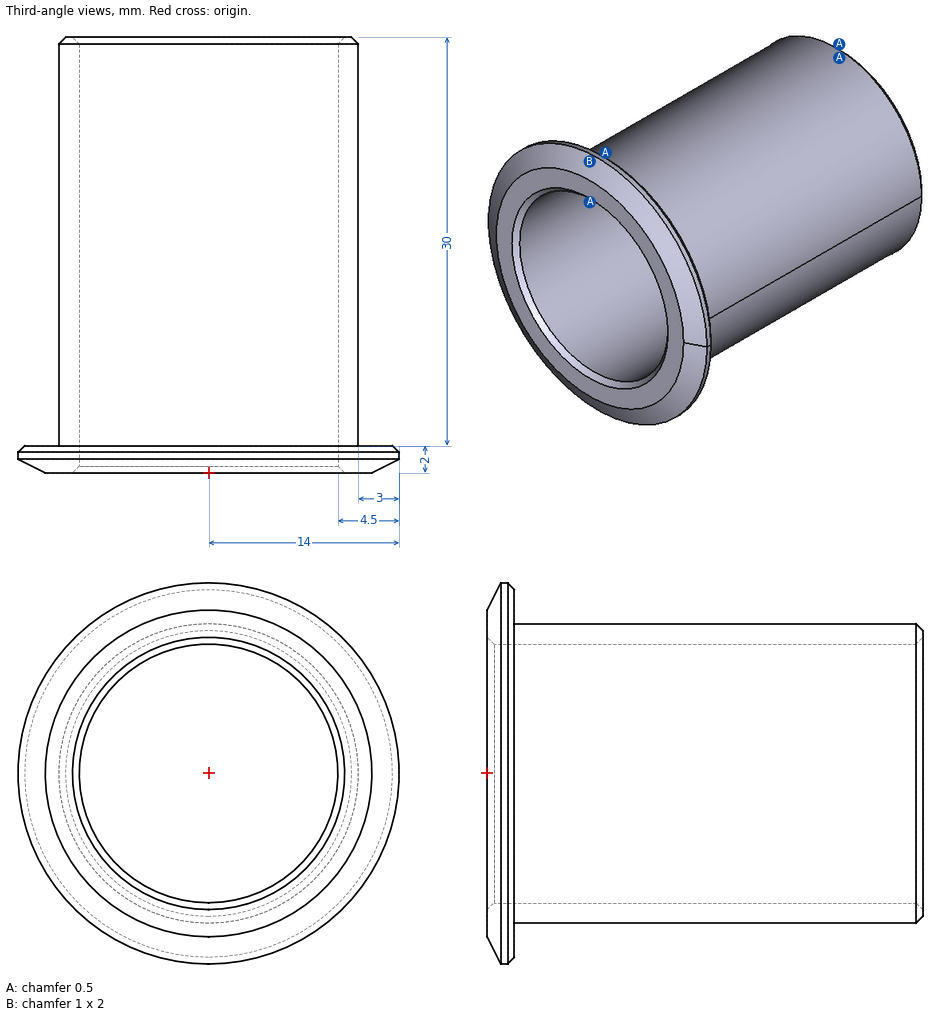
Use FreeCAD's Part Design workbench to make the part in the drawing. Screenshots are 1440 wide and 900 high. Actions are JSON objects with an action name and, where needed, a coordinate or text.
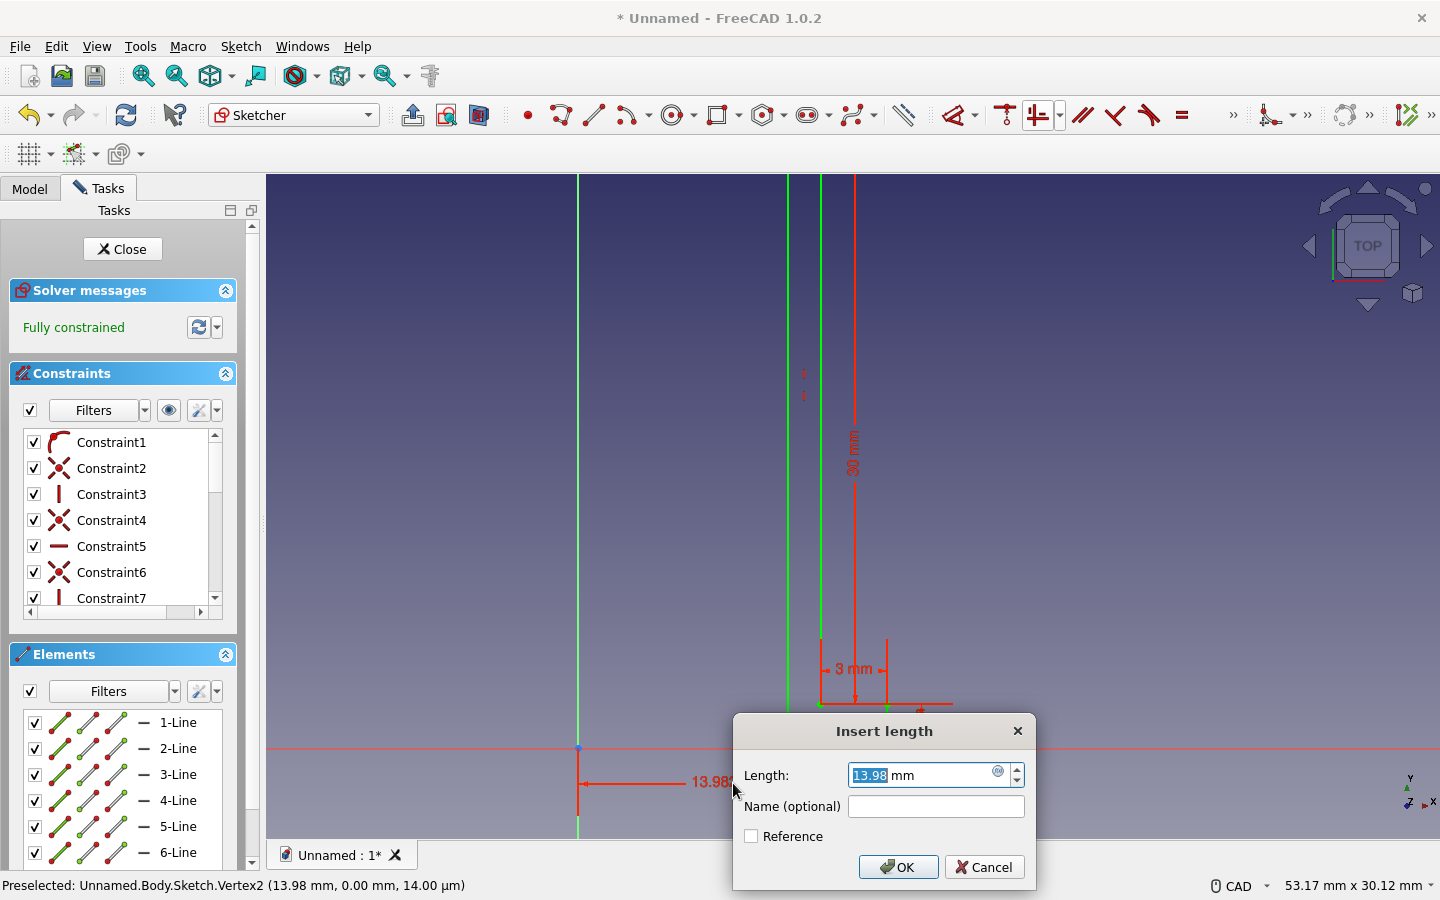
{"action": "type", "text": "14"}
{"action": "key", "text": "Return"}
{"action": "key", "text": "Escape"}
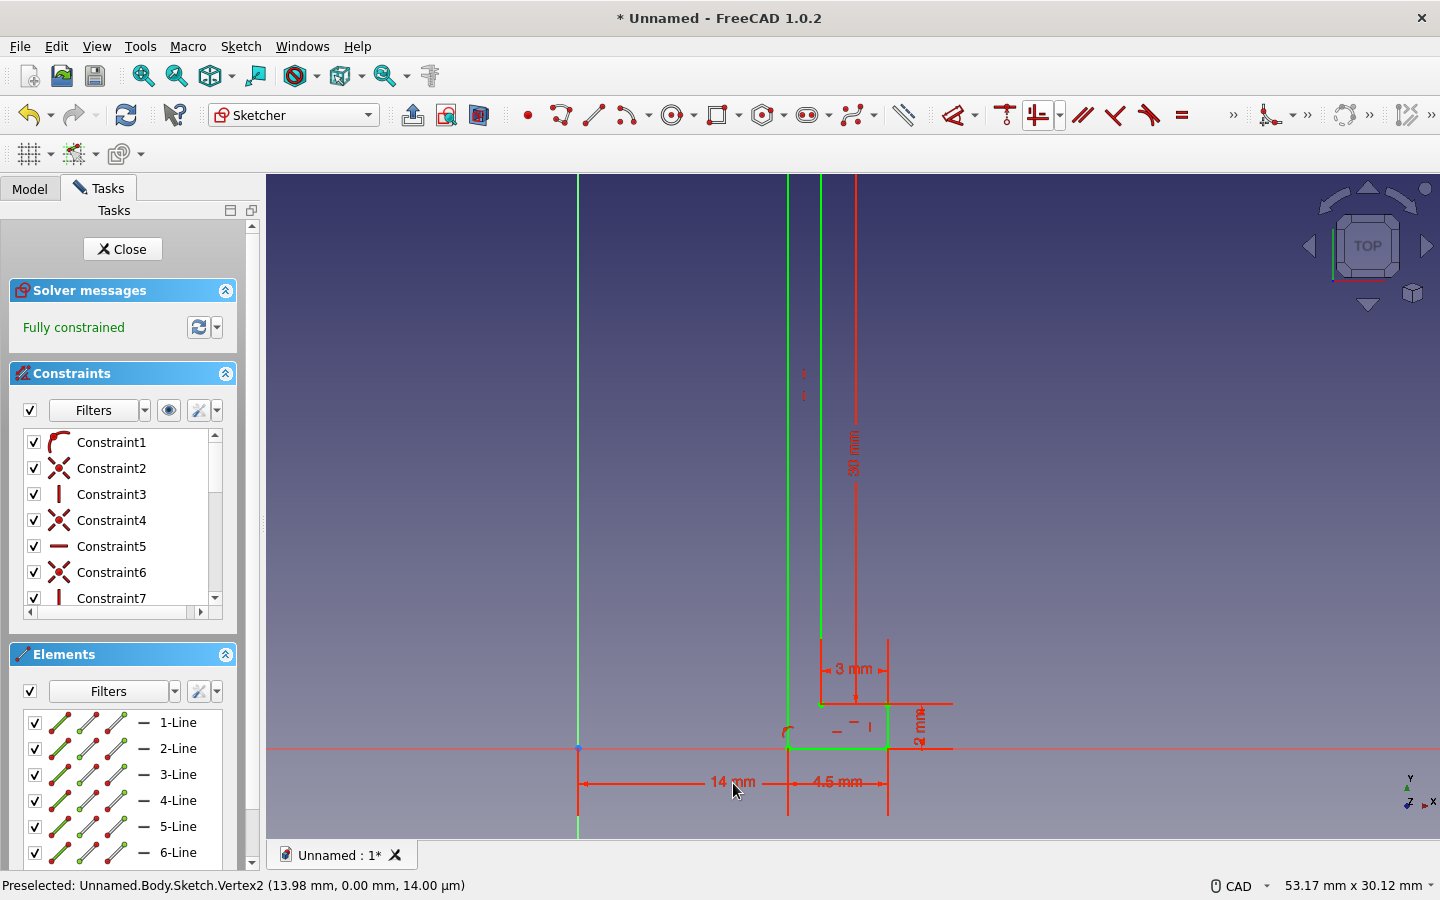
{"action": "left_click", "coordinate": [123, 249]}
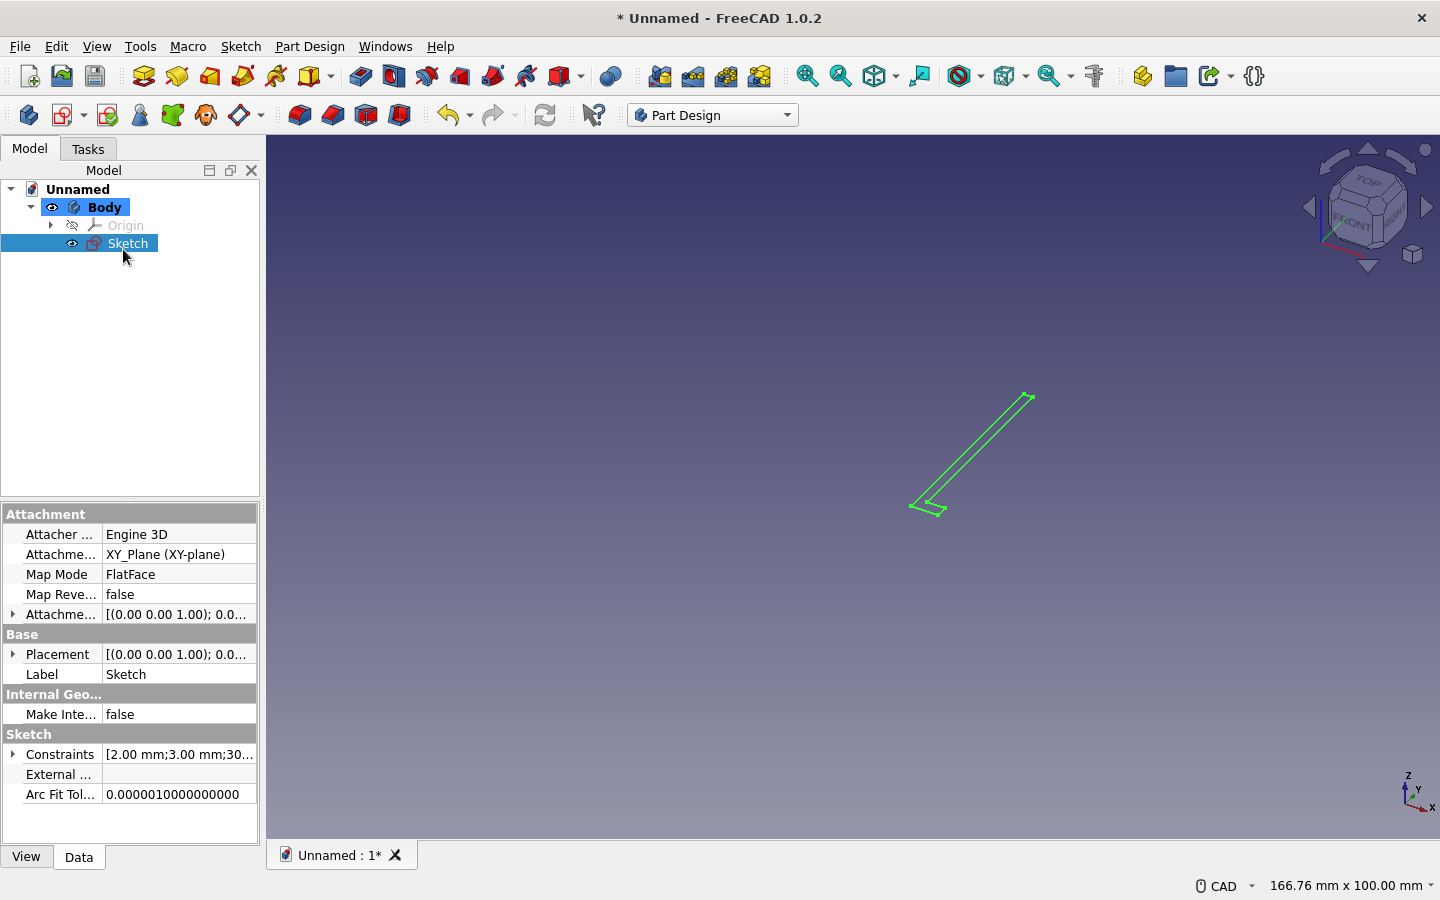
{"action": "left_click", "coordinate": [177, 76]}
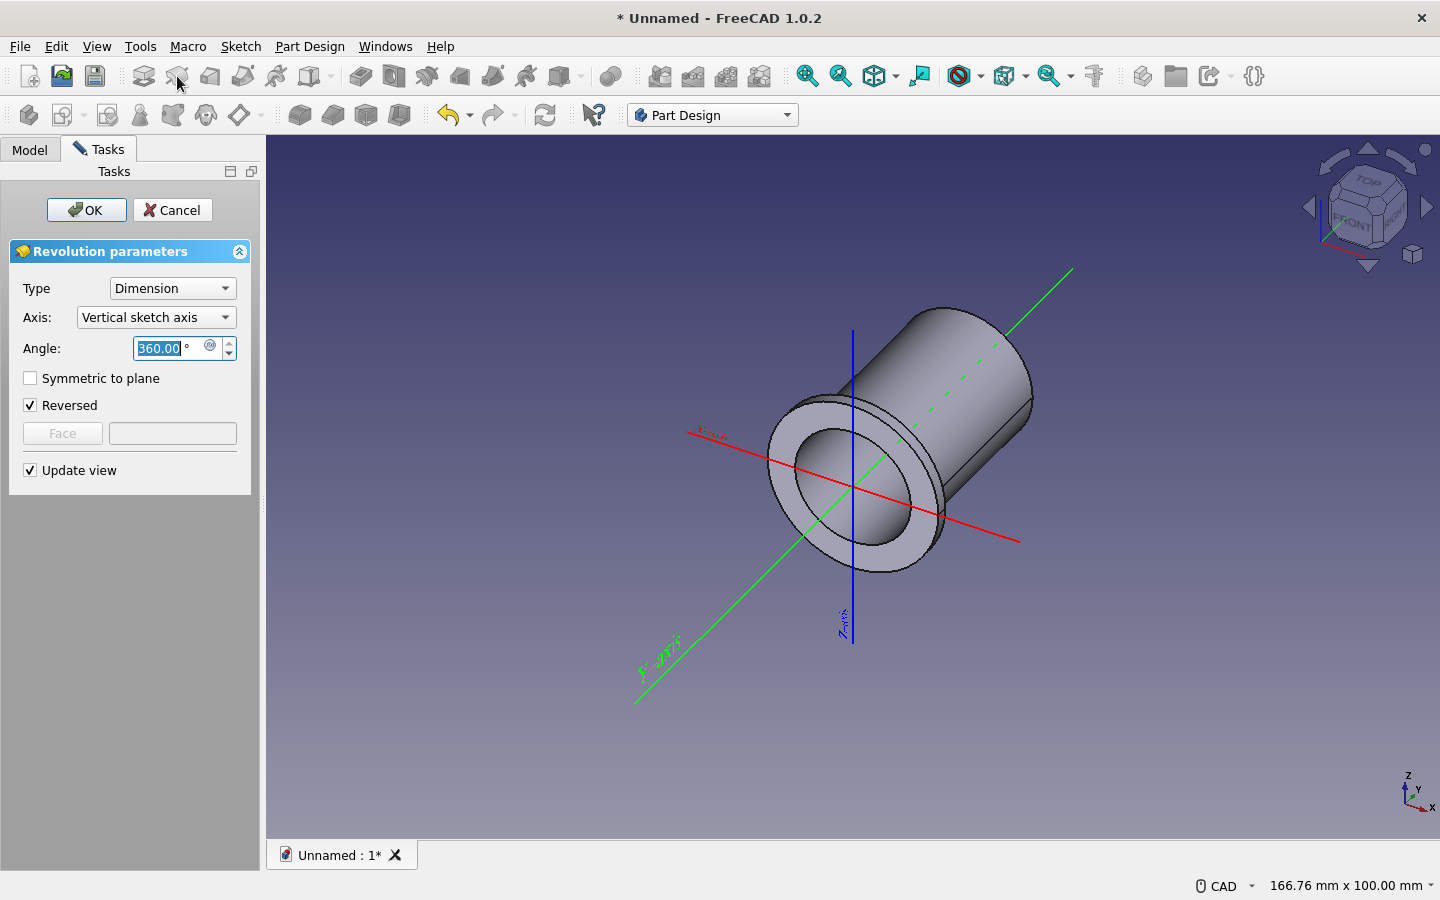
{"action": "left_click", "coordinate": [87, 210]}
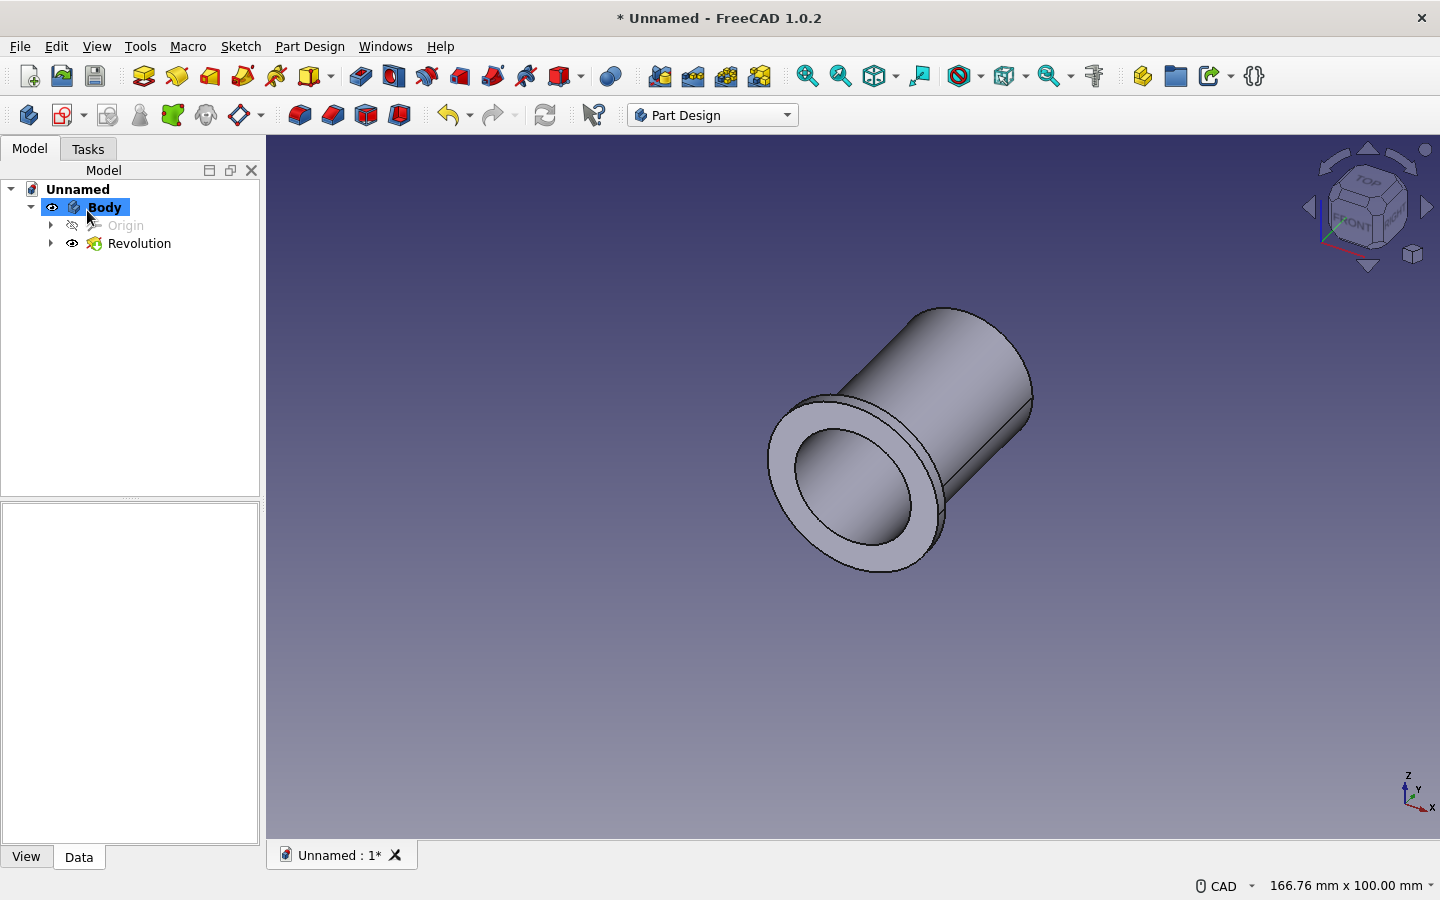
{"action": "left_click", "coordinate": [795, 467]}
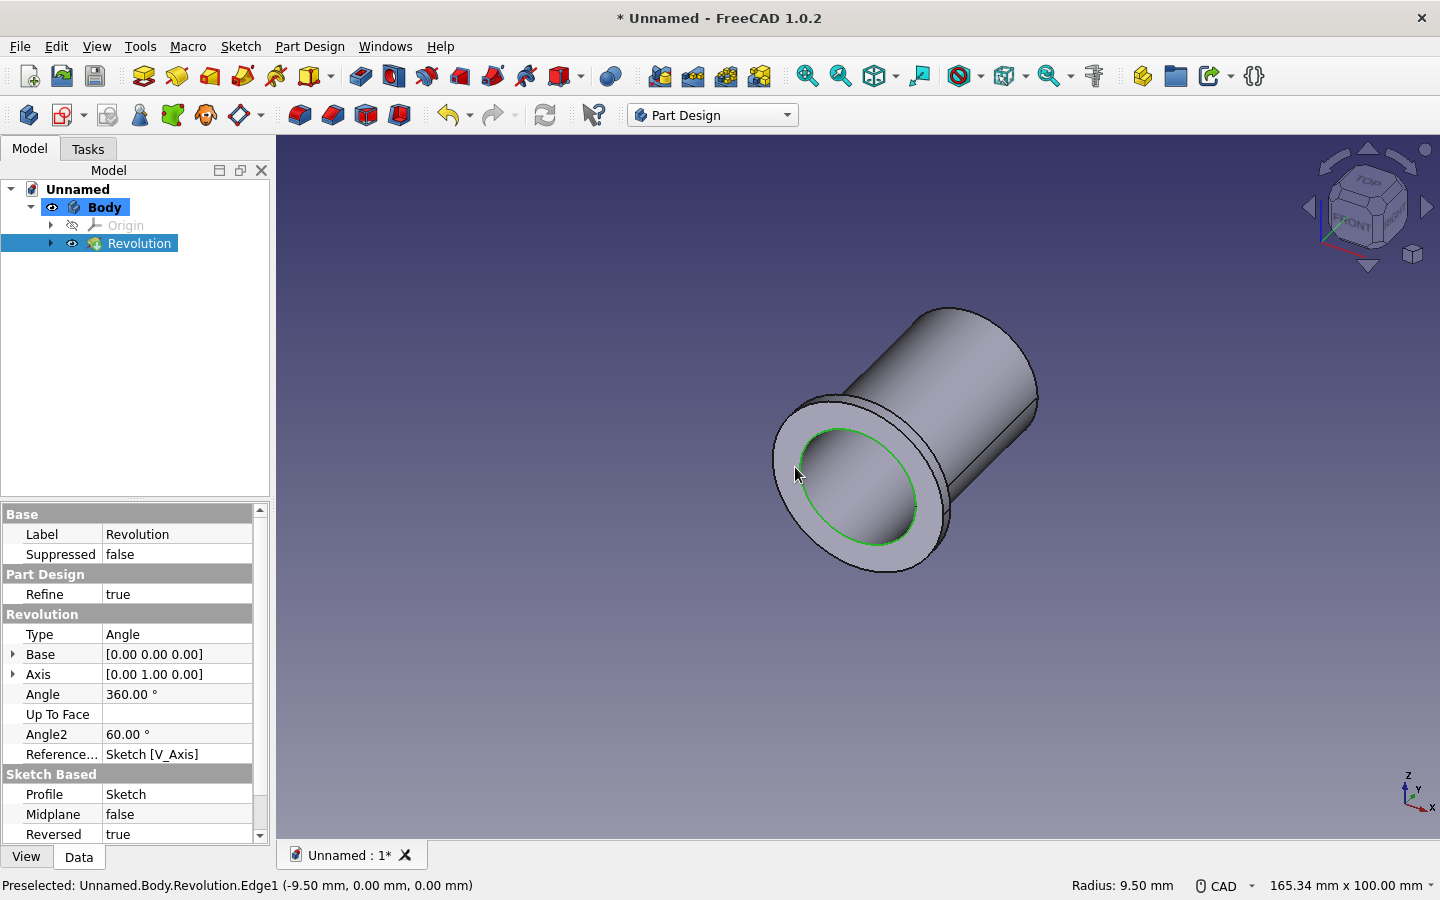
{"action": "key", "text": "0"}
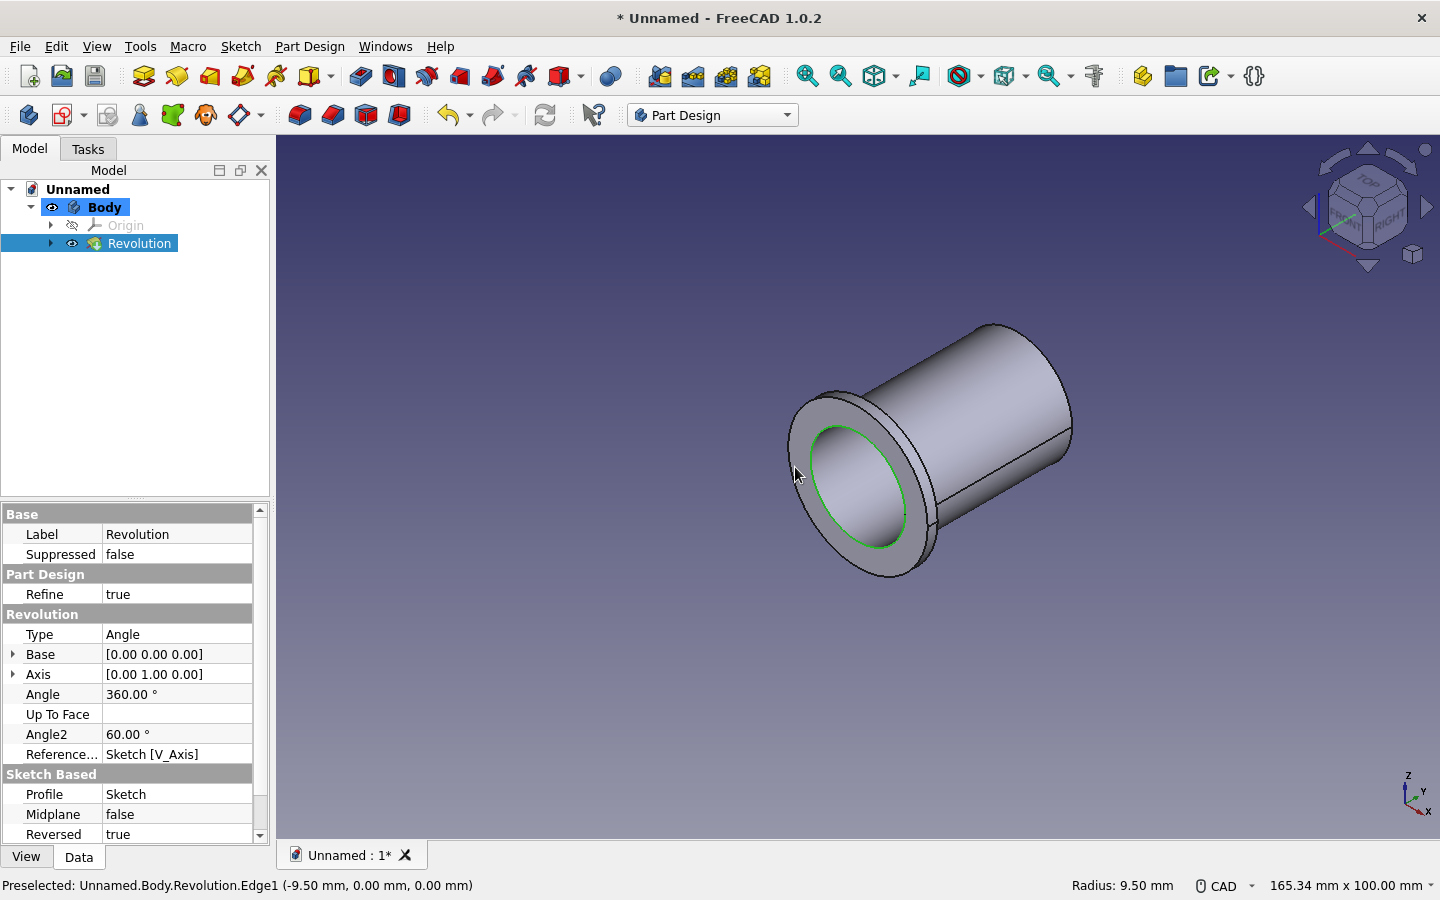
{"action": "key", "text": "2"}